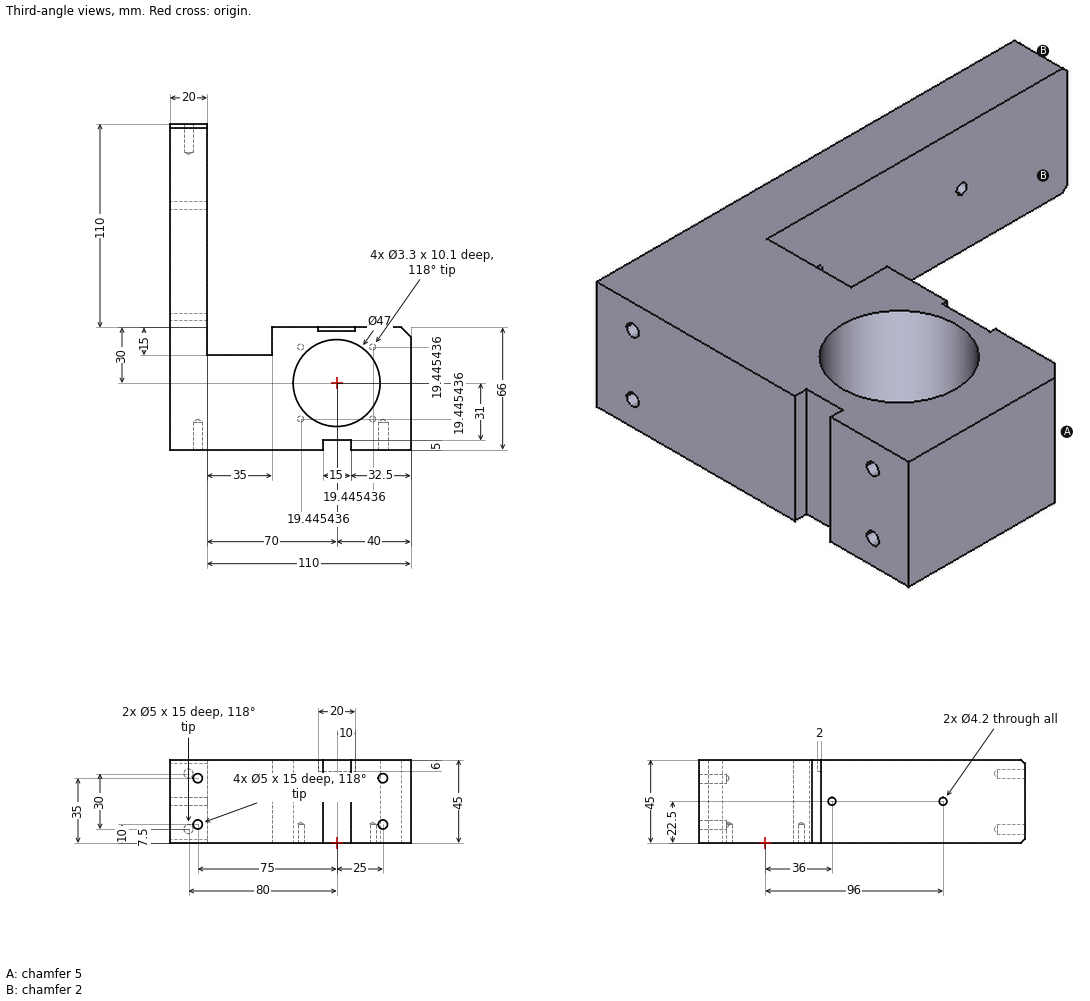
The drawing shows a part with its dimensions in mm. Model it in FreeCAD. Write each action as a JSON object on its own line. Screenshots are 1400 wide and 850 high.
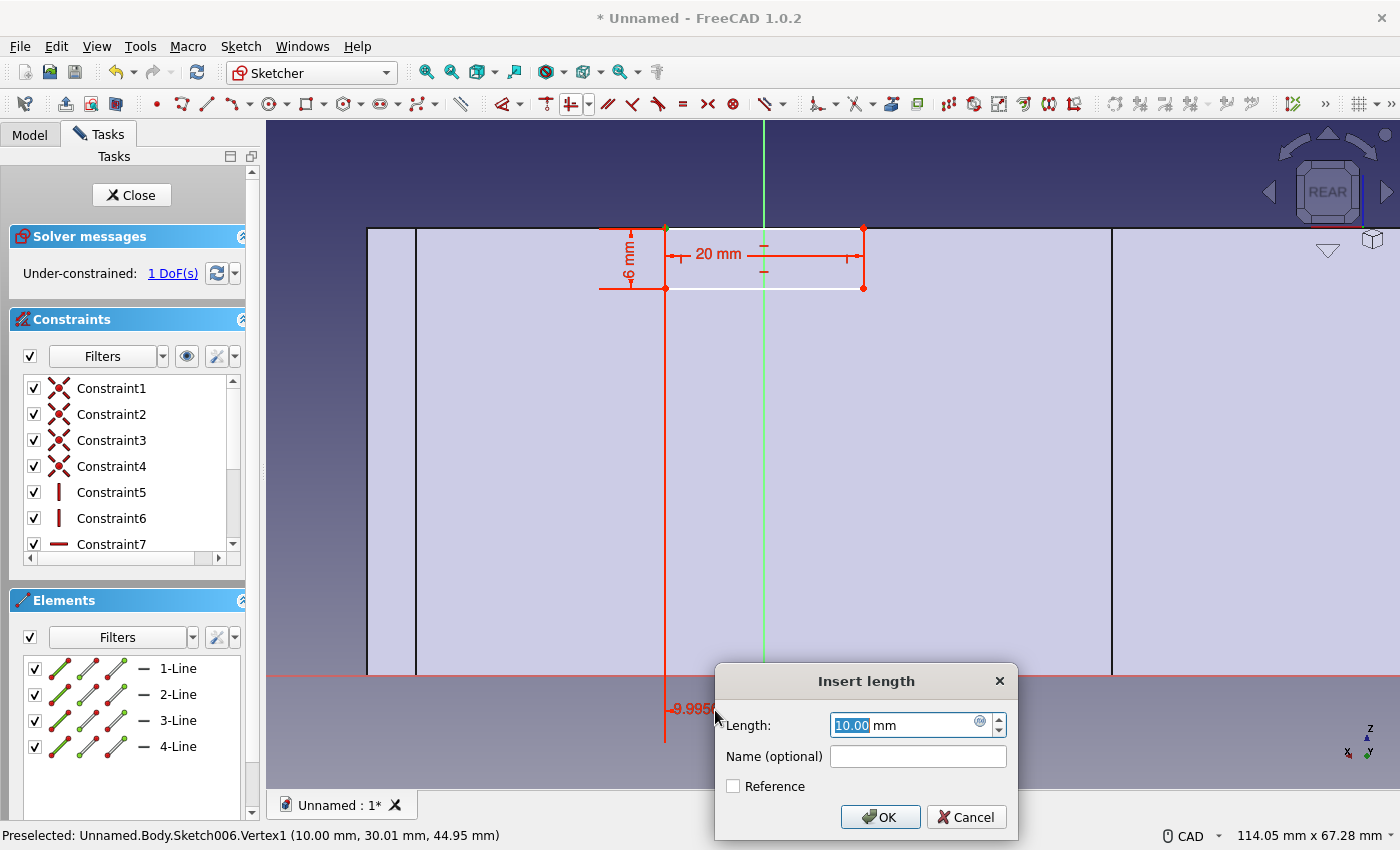
{"action": "type", "text": "10"}
{"action": "key", "text": "Return"}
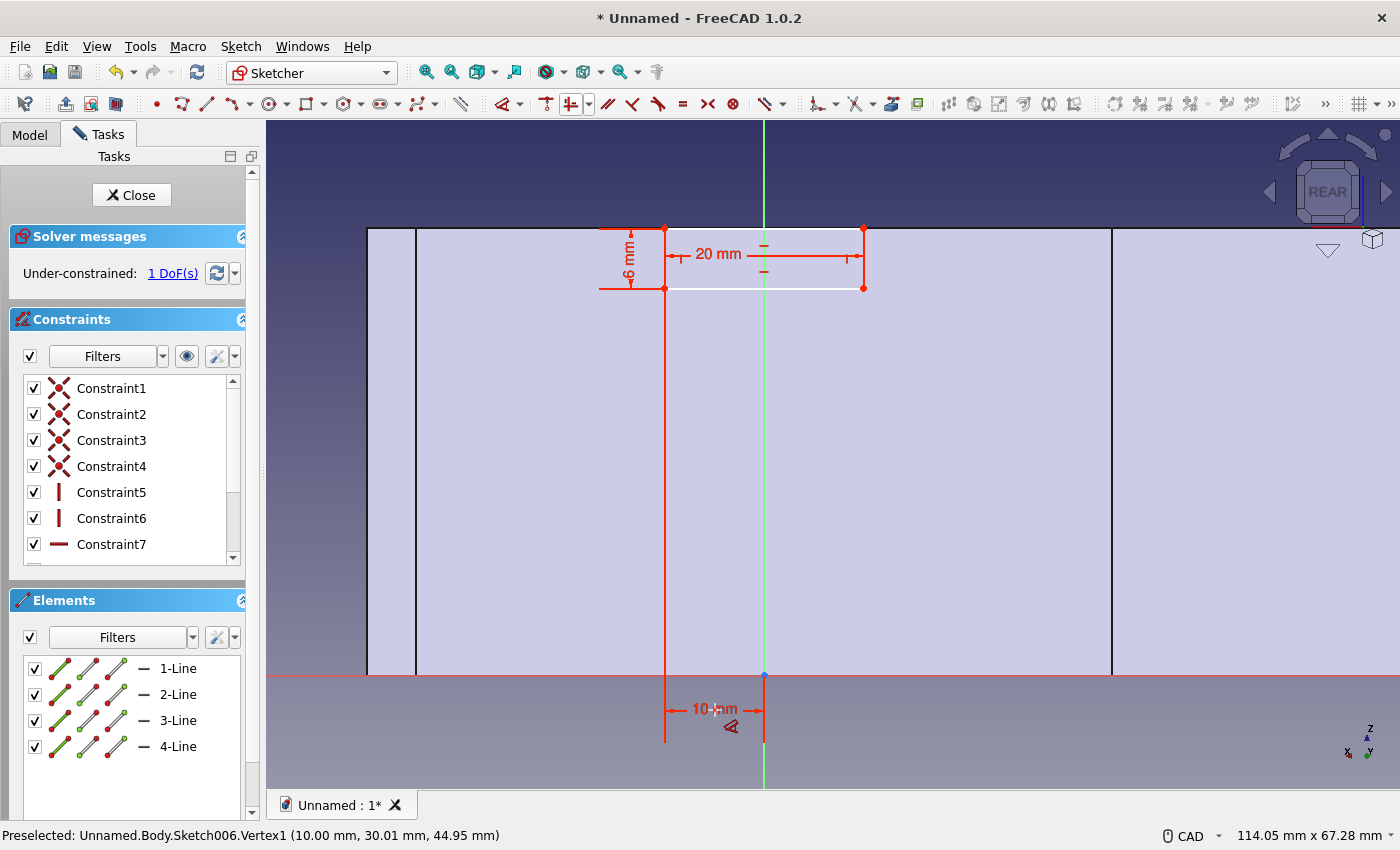
{"action": "left_click", "coordinate": [665, 229]}
{"action": "left_click", "coordinate": [631, 452]}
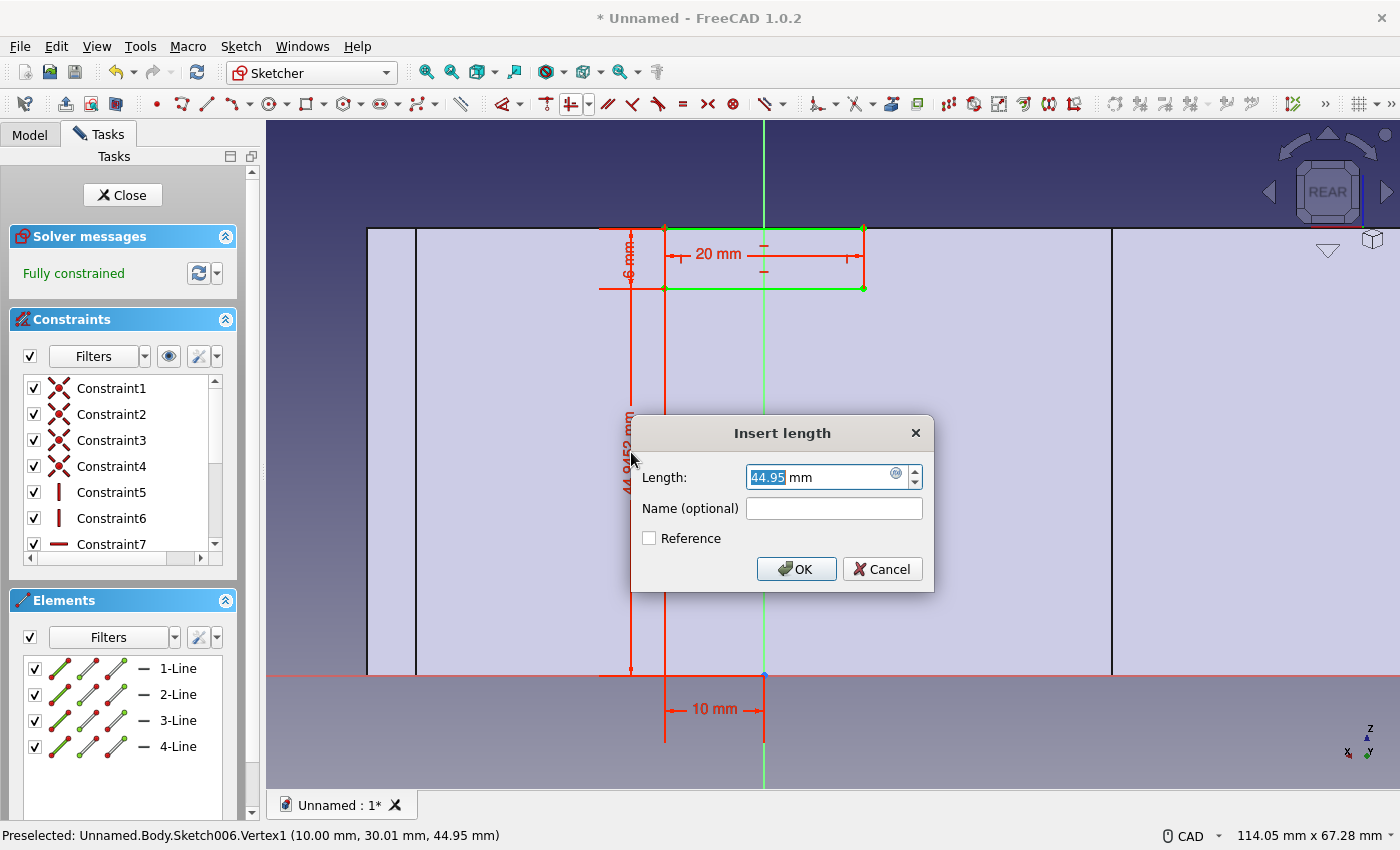
{"action": "type", "text": "45"}
{"action": "key", "text": "Return"}
{"action": "key", "text": "Escape"}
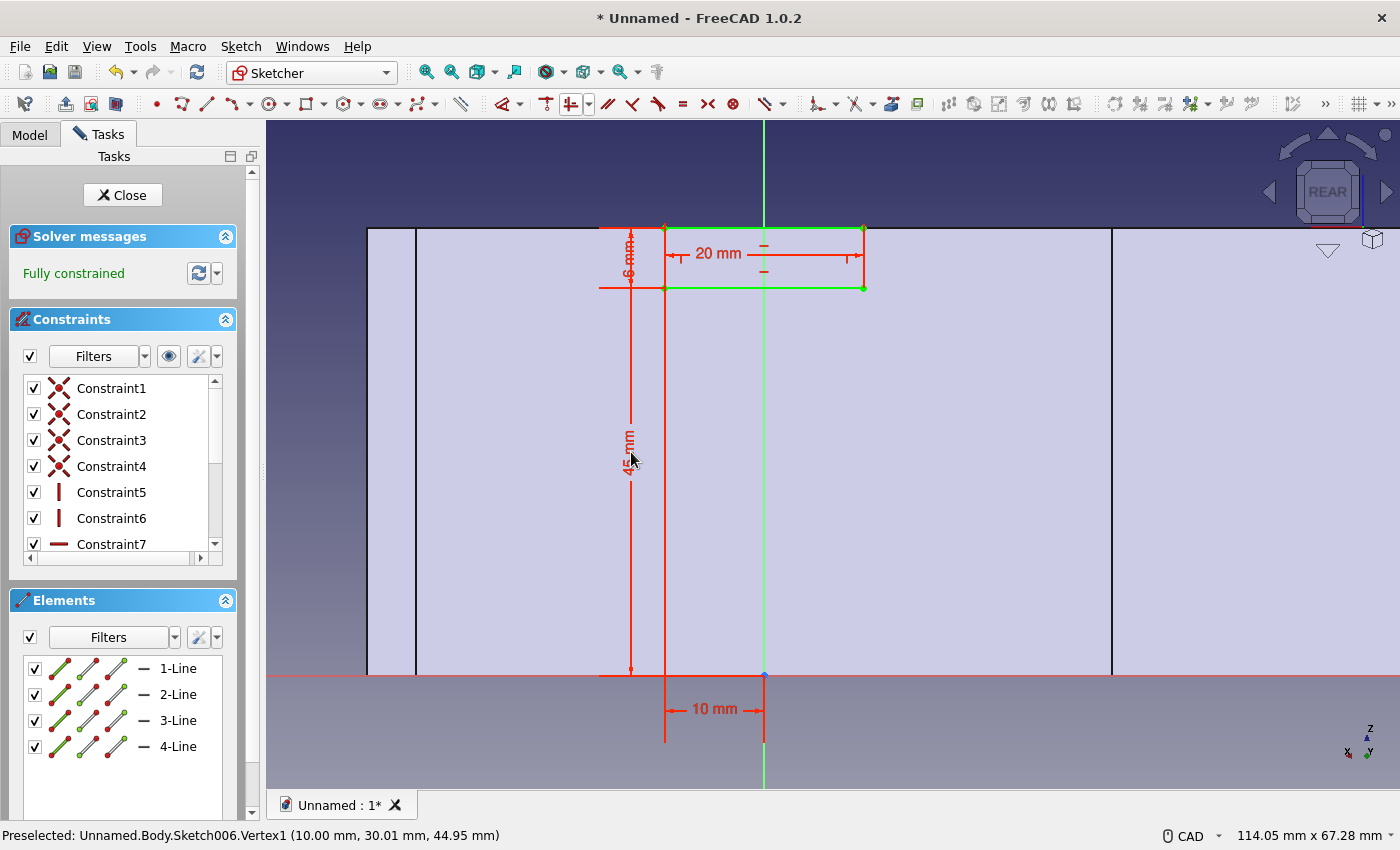
{"action": "left_click", "coordinate": [123, 195]}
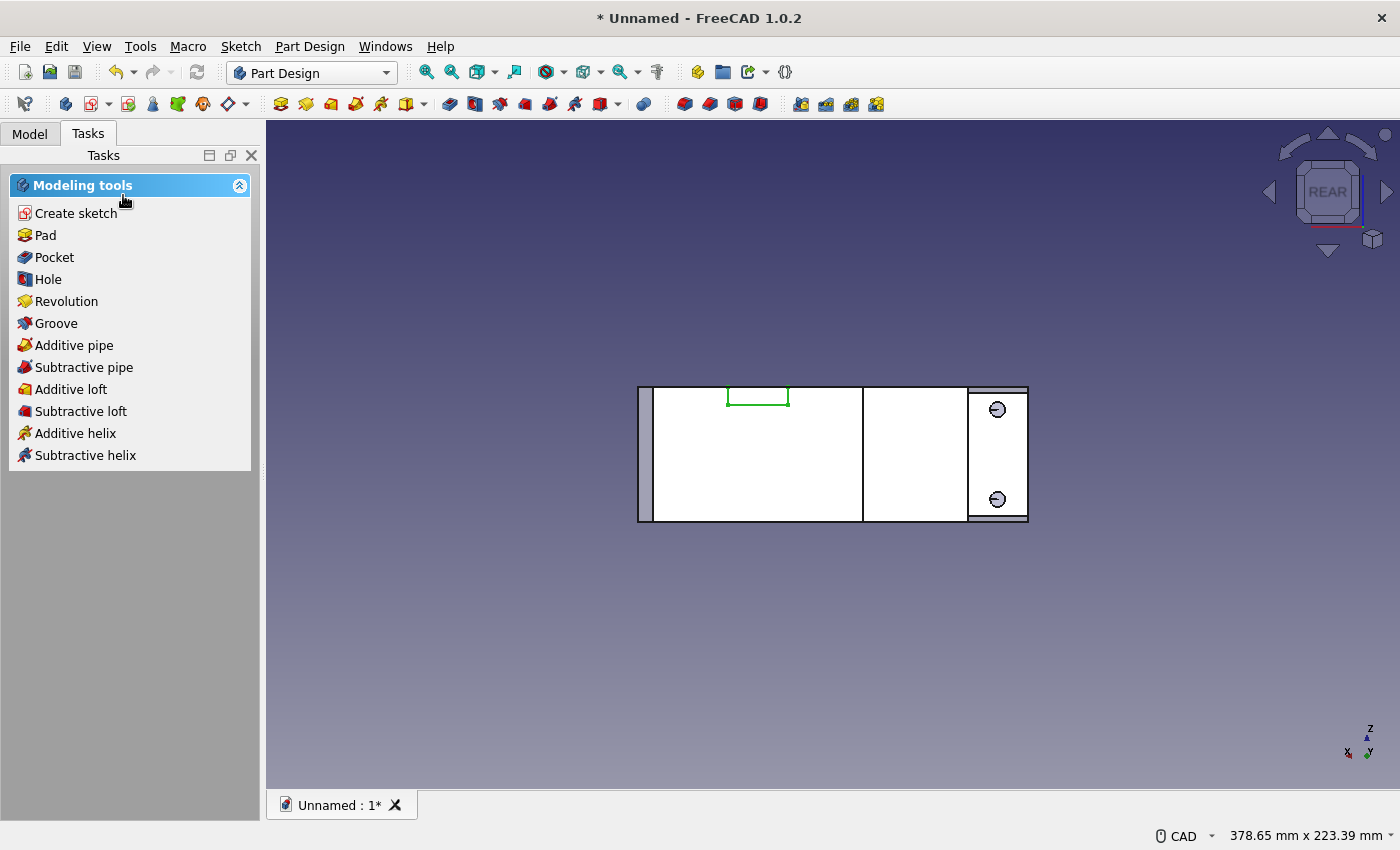
{"action": "left_click", "coordinate": [450, 104]}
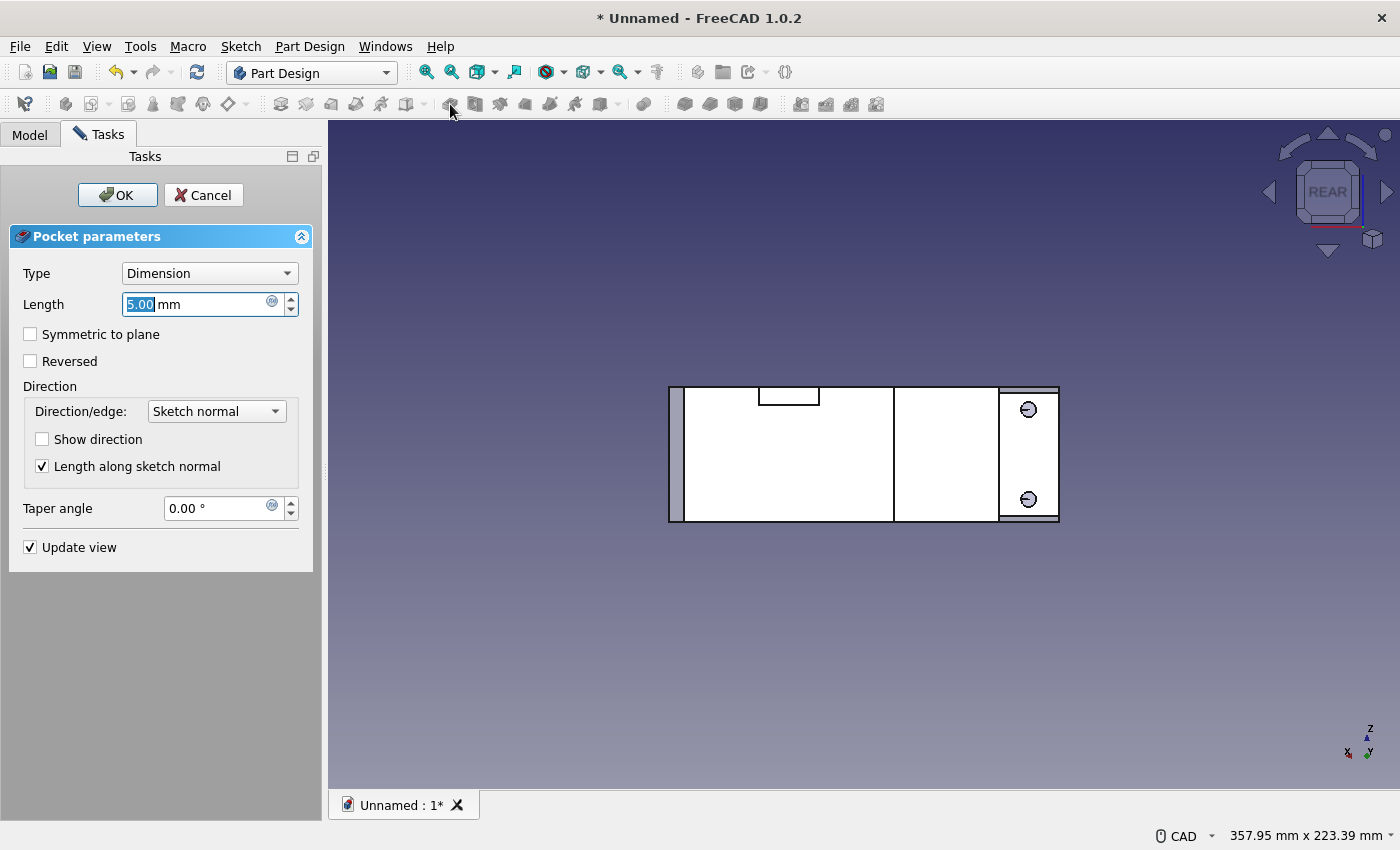
{"action": "type", "text": "2"}
{"action": "key", "text": "Tab"}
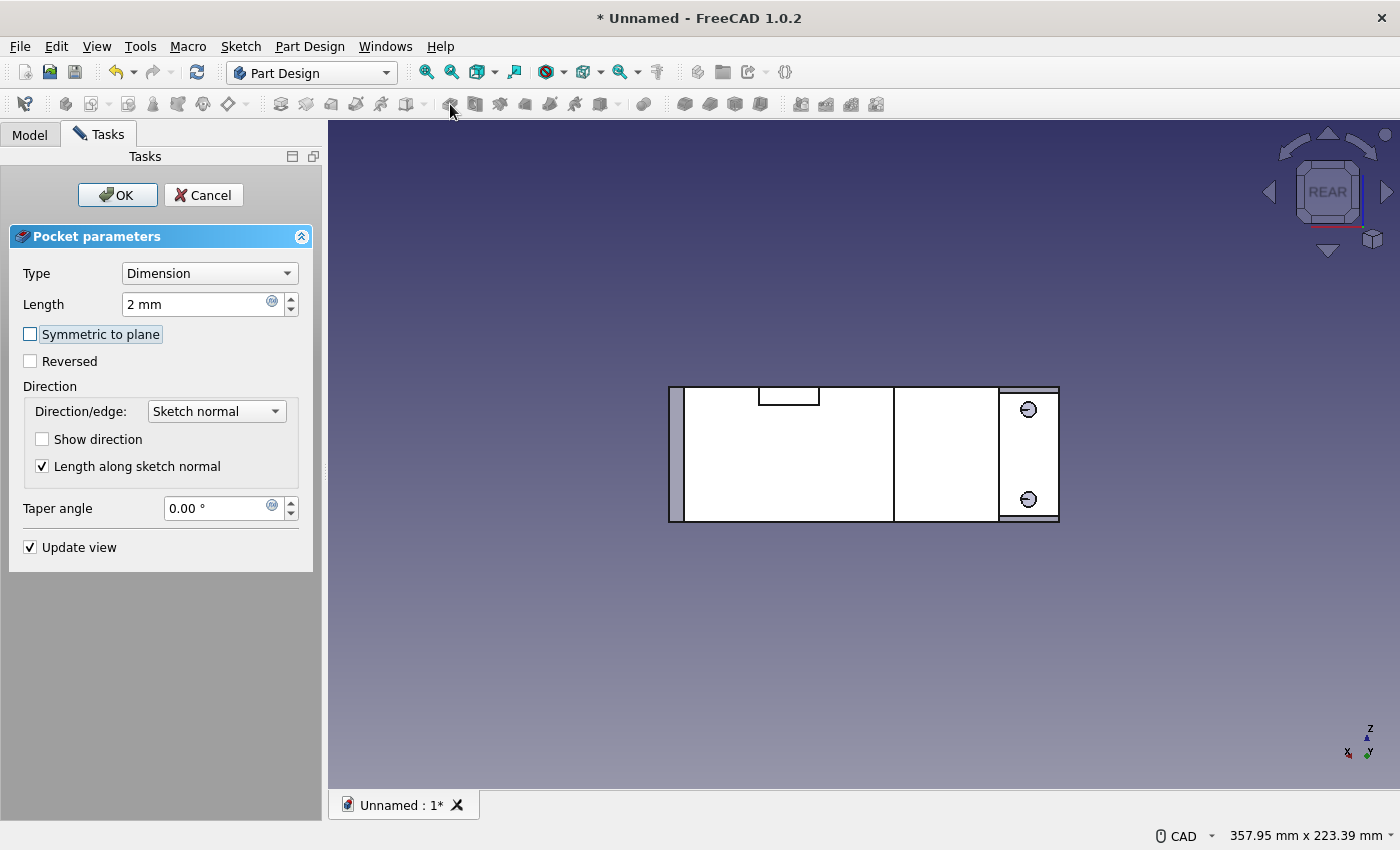
{"action": "left_click", "coordinate": [118, 195]}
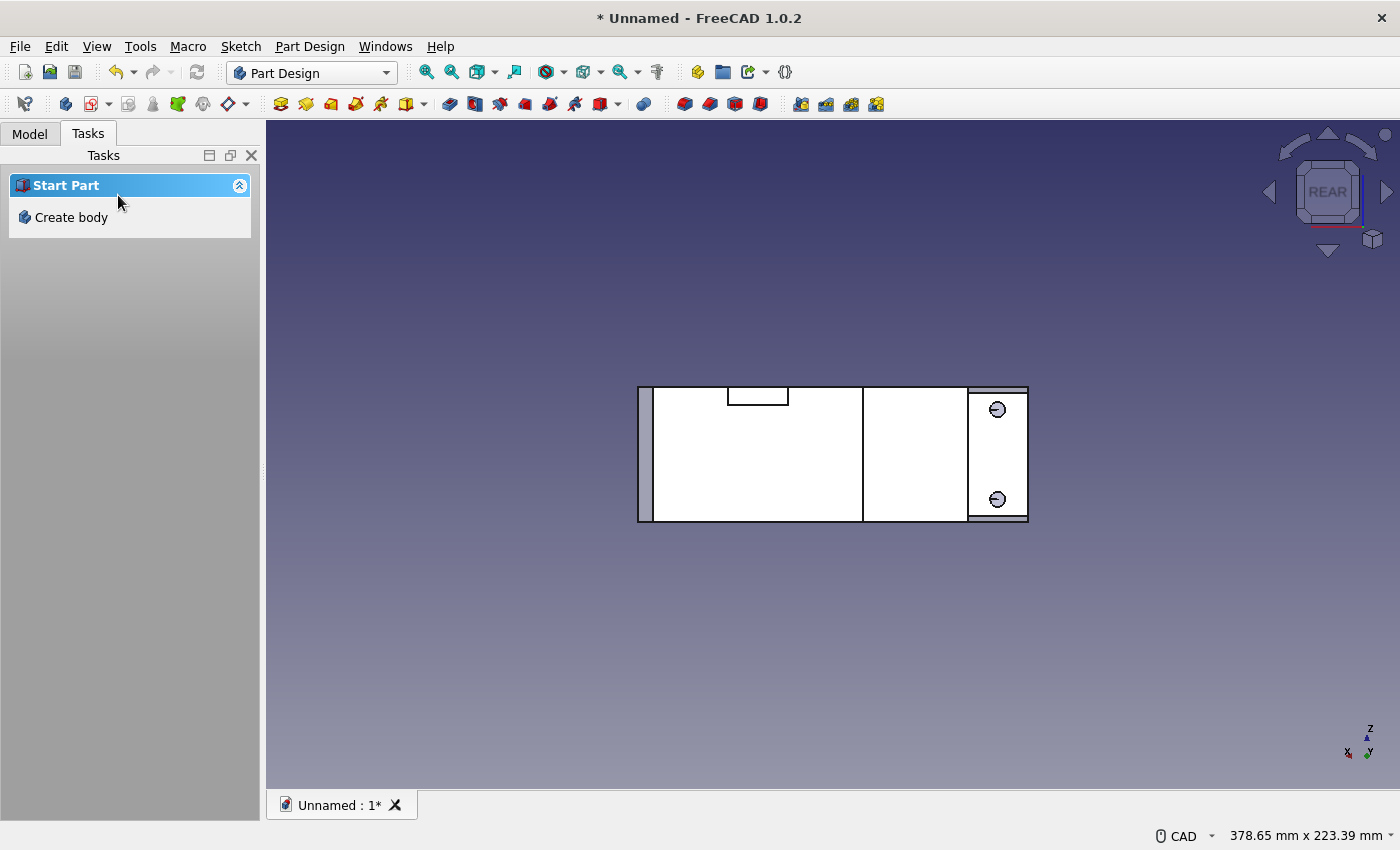
{"action": "key", "text": "0"}